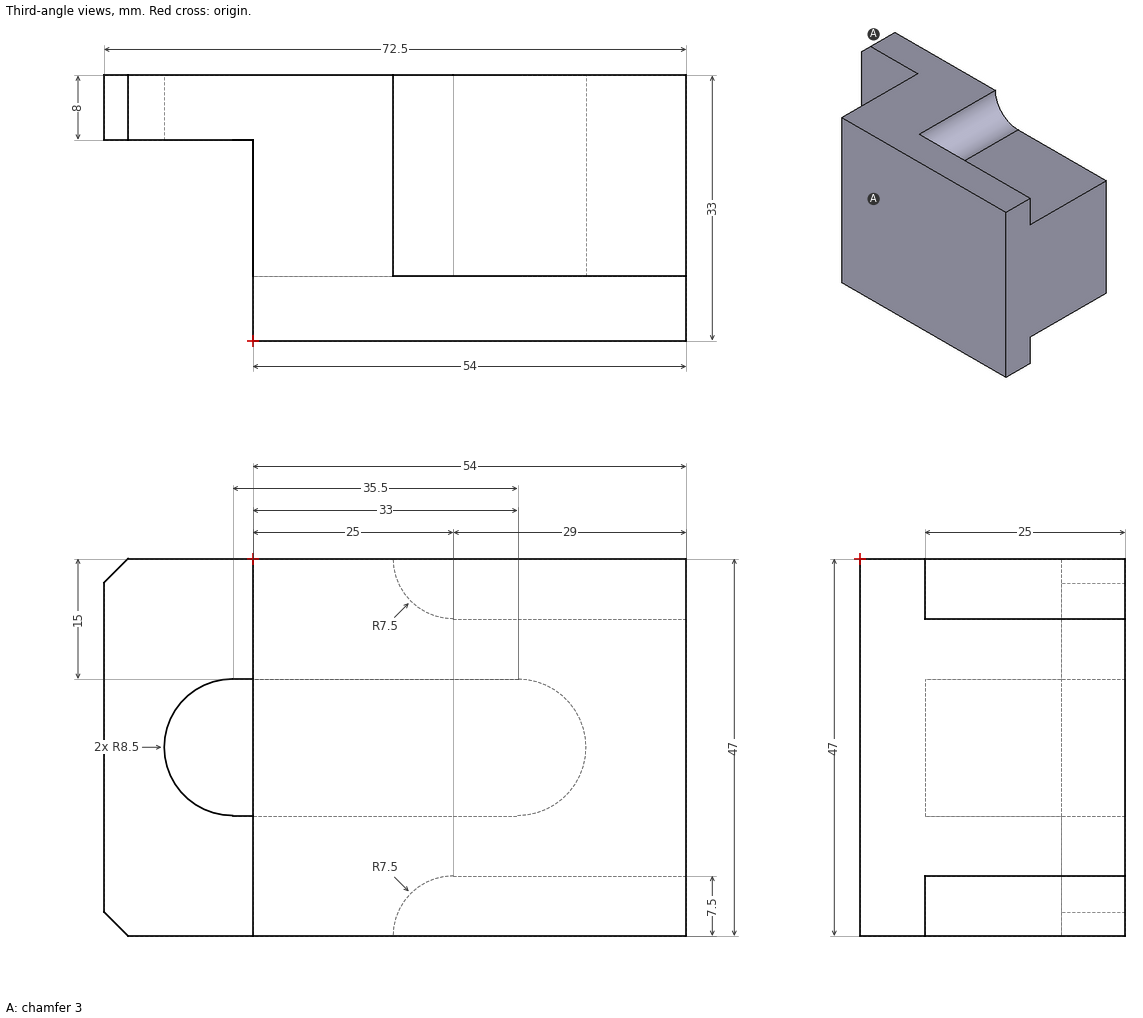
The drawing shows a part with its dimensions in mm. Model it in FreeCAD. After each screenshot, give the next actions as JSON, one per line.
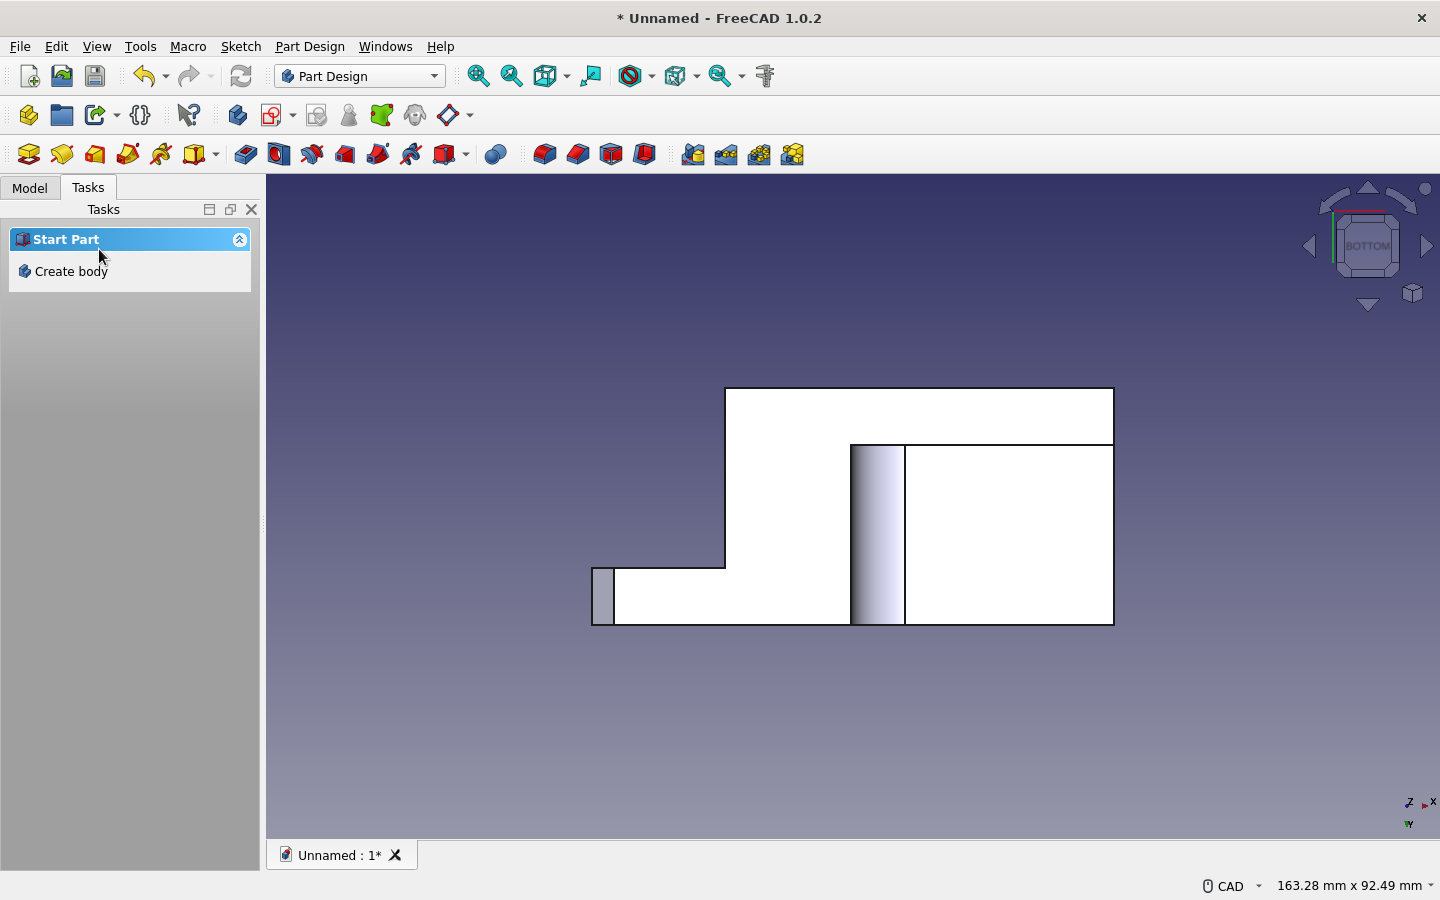
{"action": "key", "text": "0"}